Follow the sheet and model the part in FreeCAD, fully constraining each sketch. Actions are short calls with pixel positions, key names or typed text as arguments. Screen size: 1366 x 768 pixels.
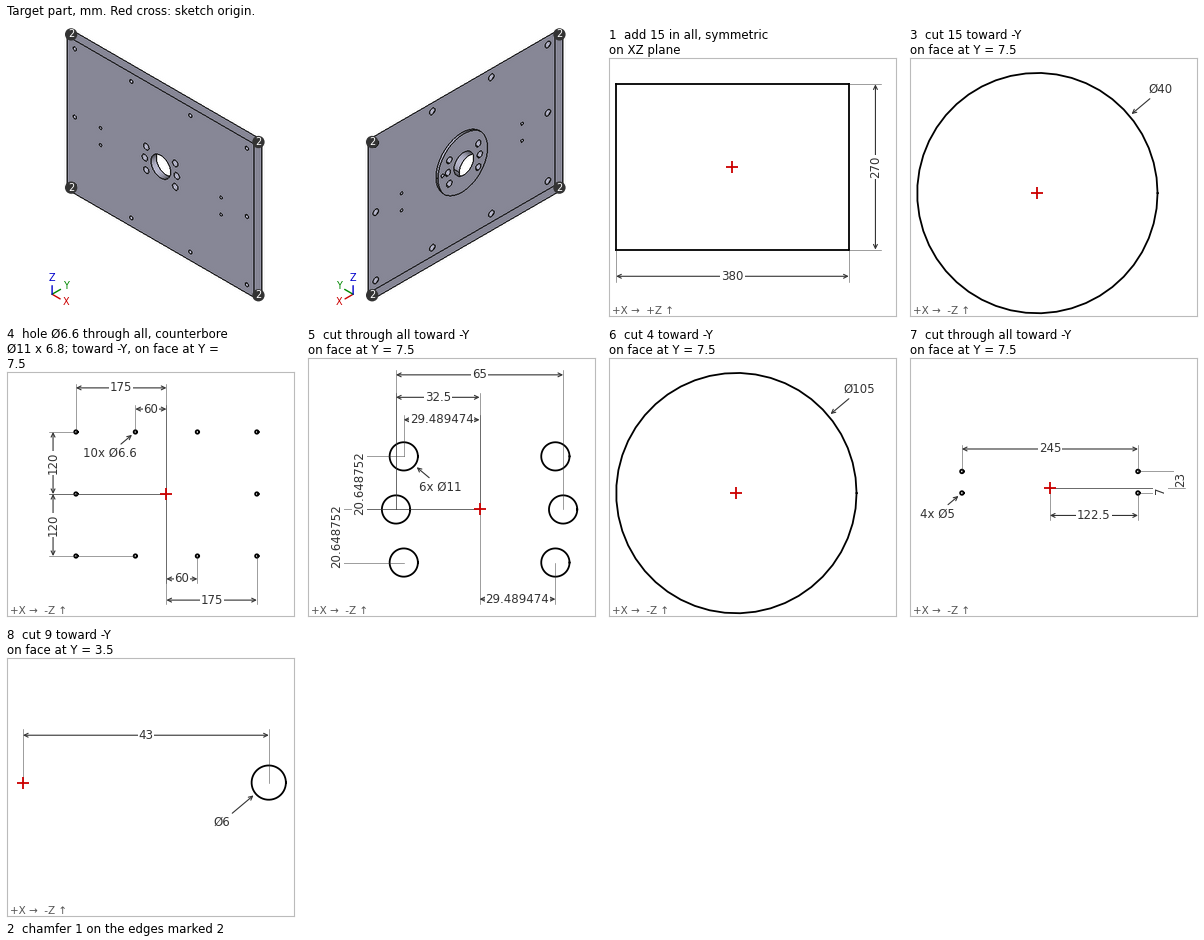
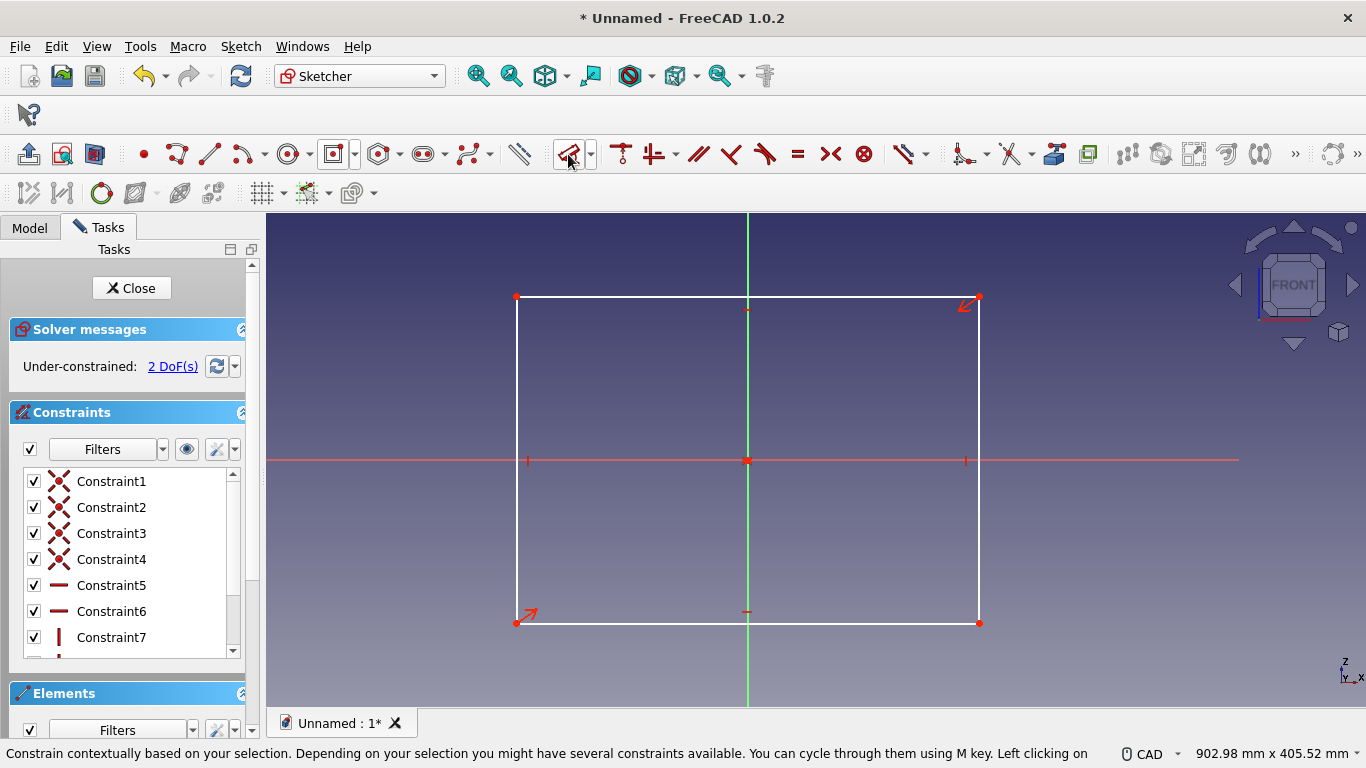
click(655, 624)
click(641, 658)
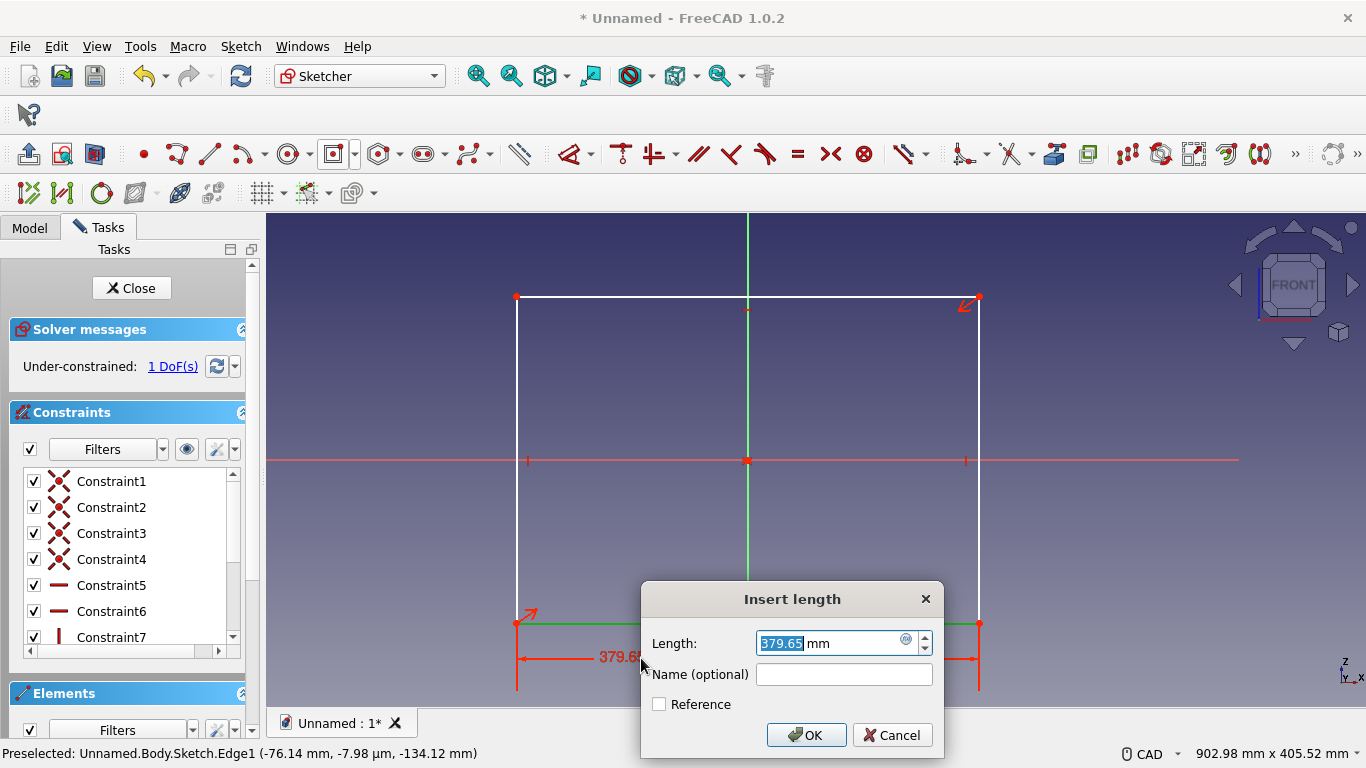
text(380)
key(Return)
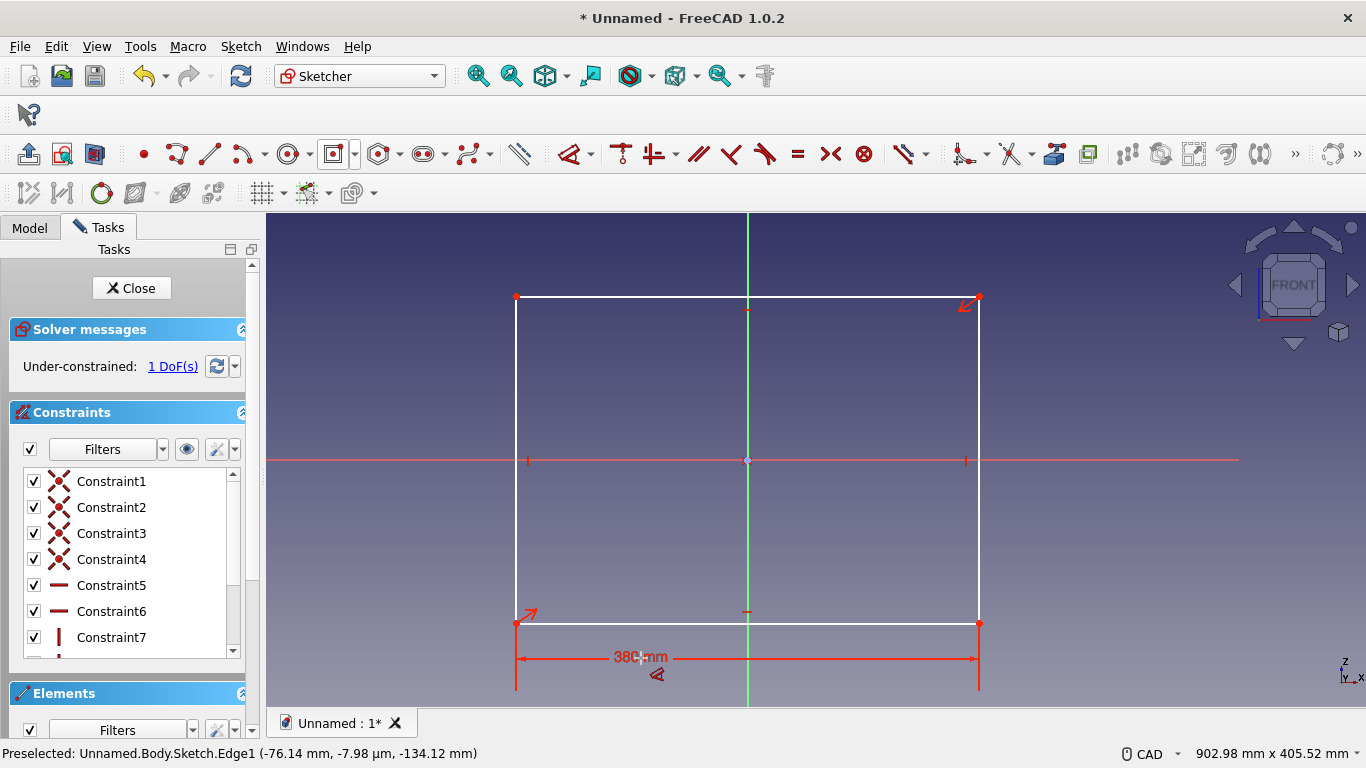
click(979, 526)
click(1013, 385)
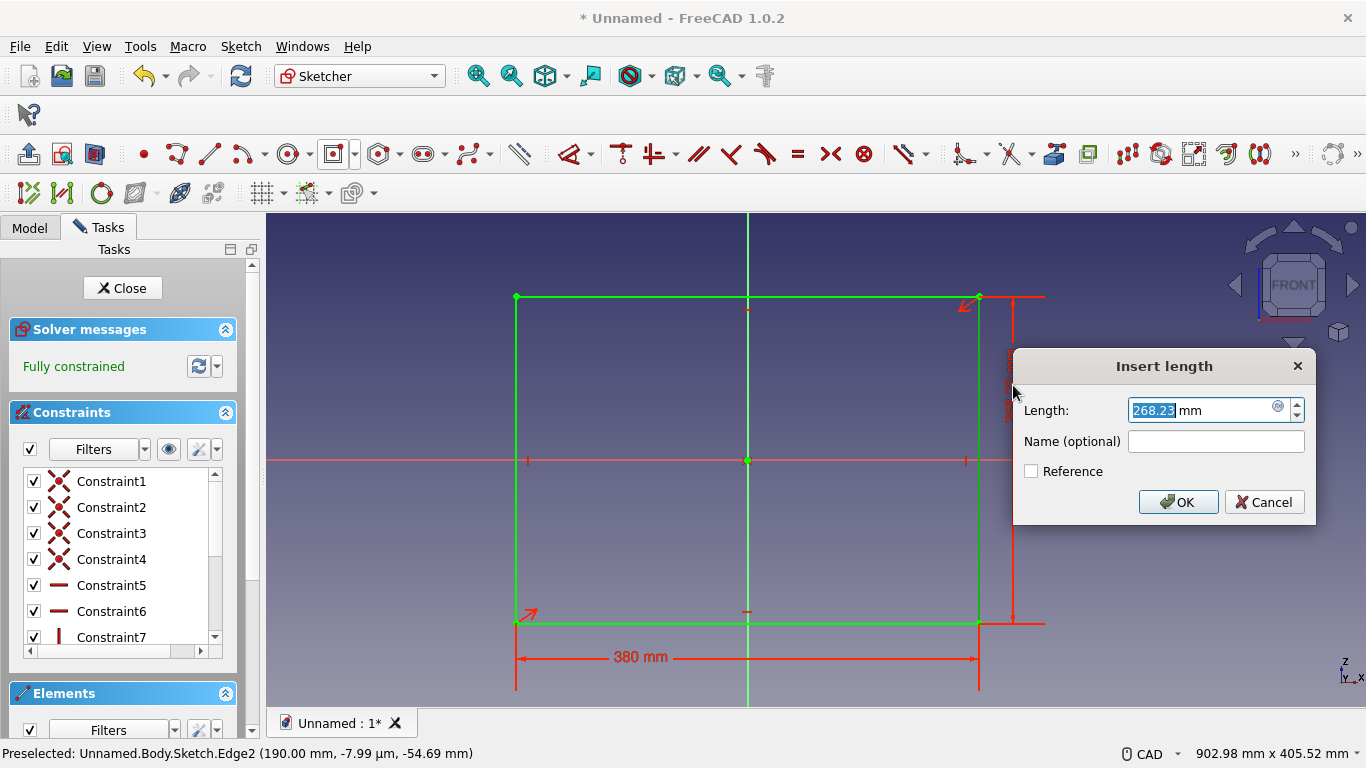
text(270)
key(Return)
key(Escape)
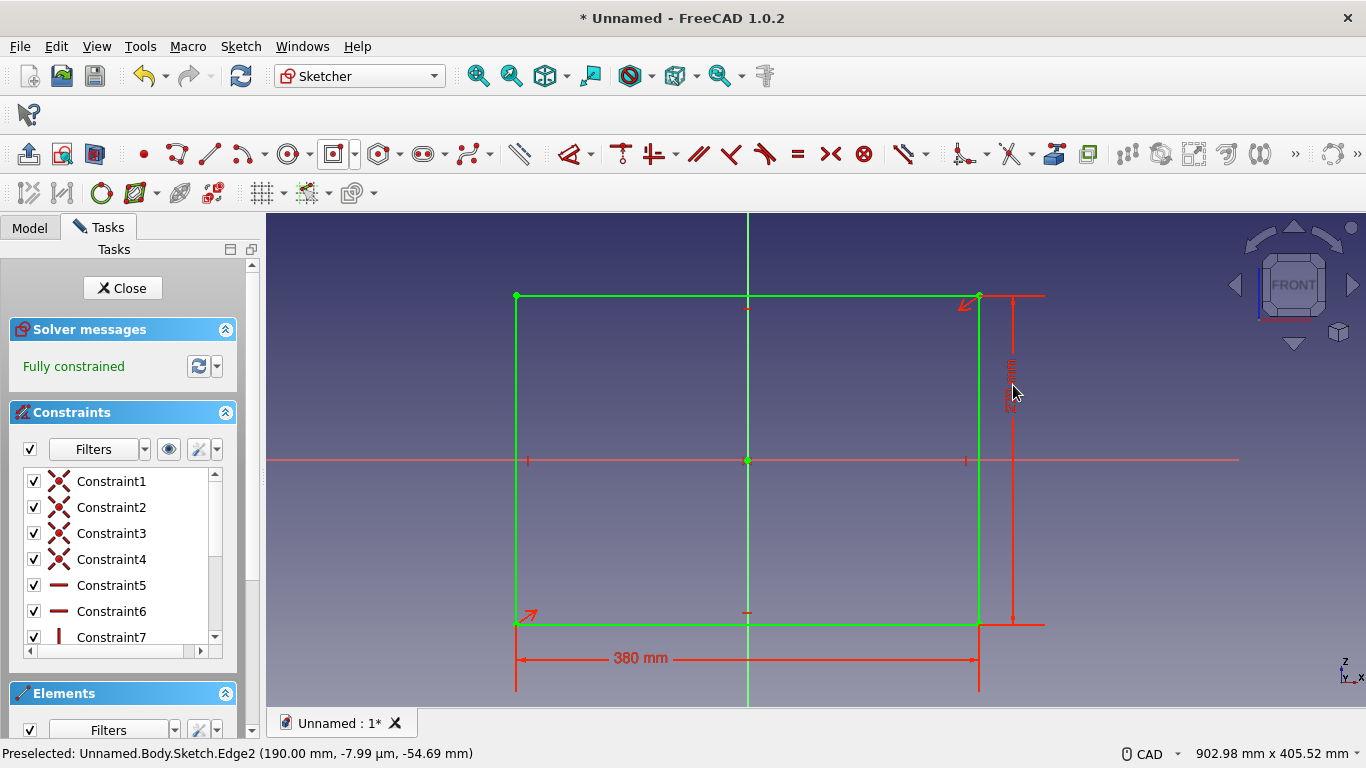
click(123, 288)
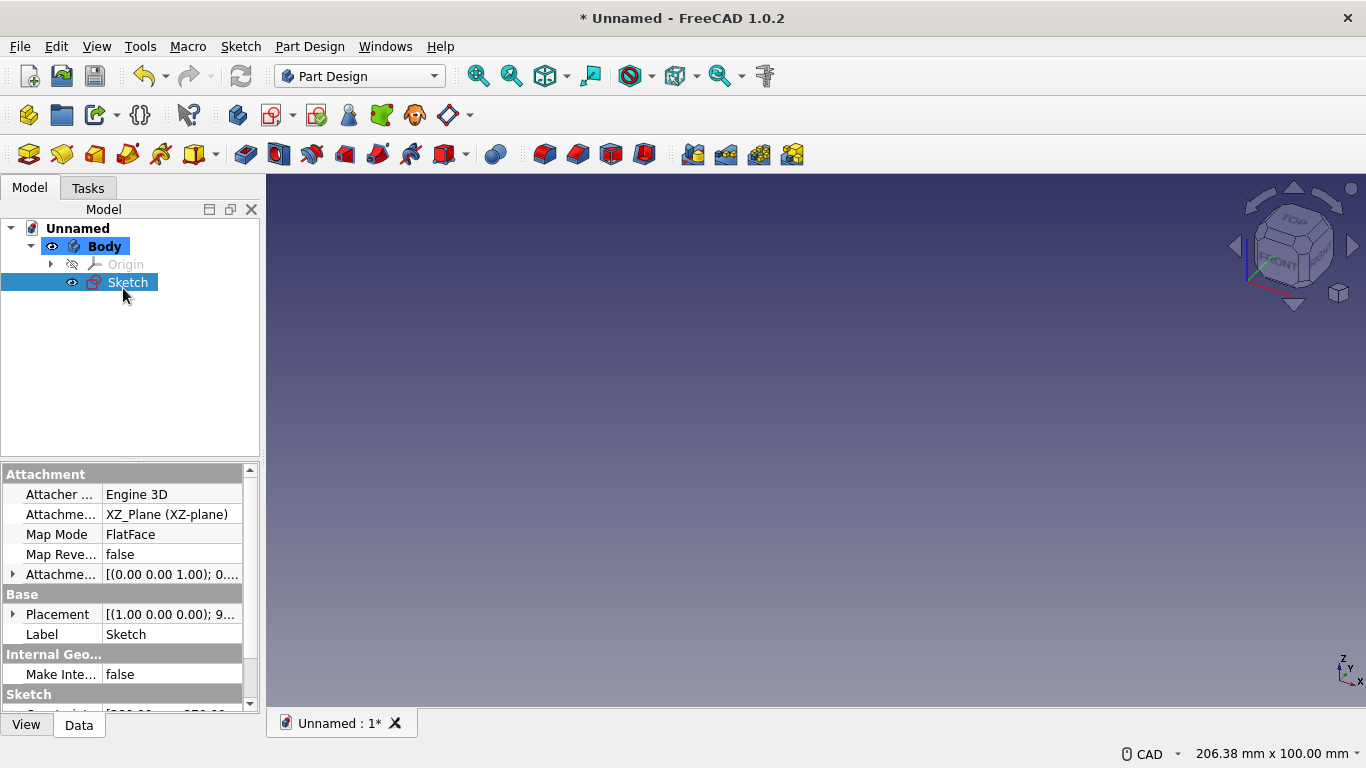
click(29, 154)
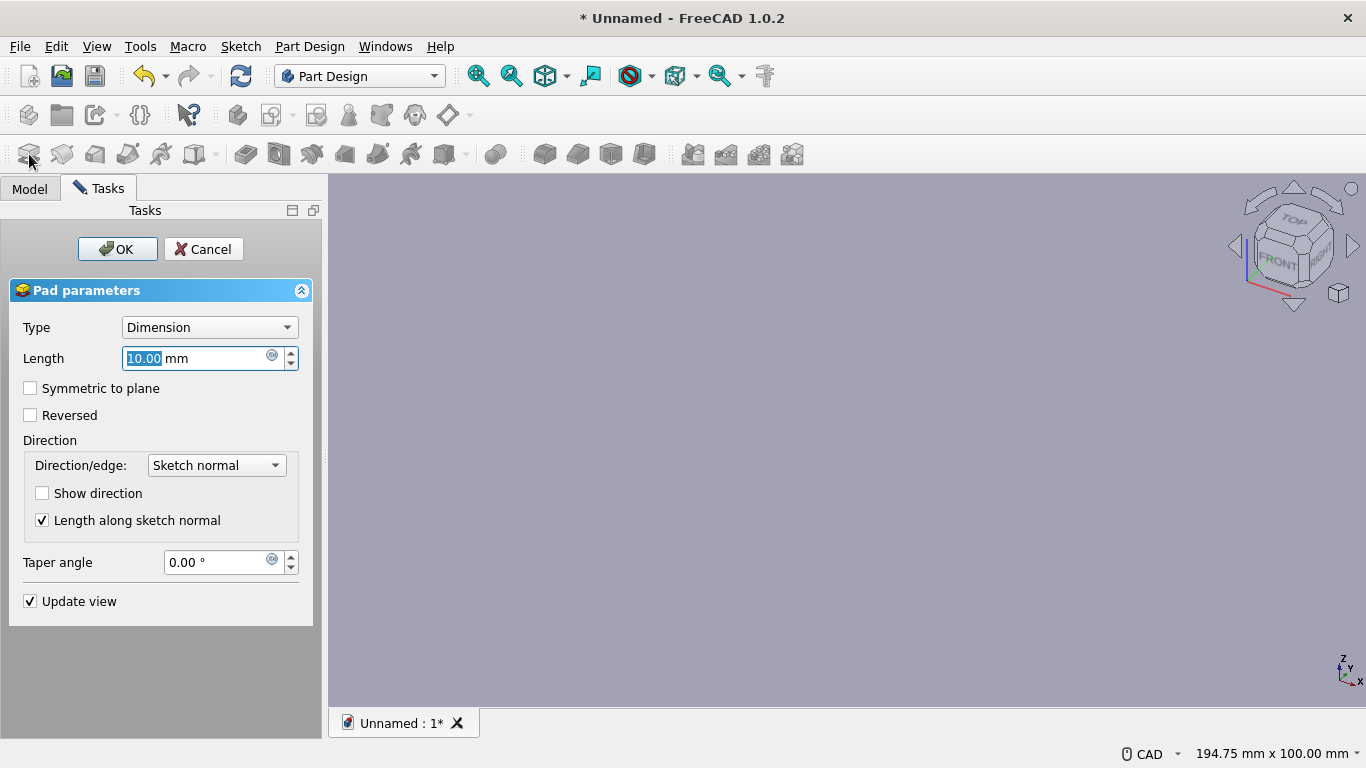
text(15)
key(Tab)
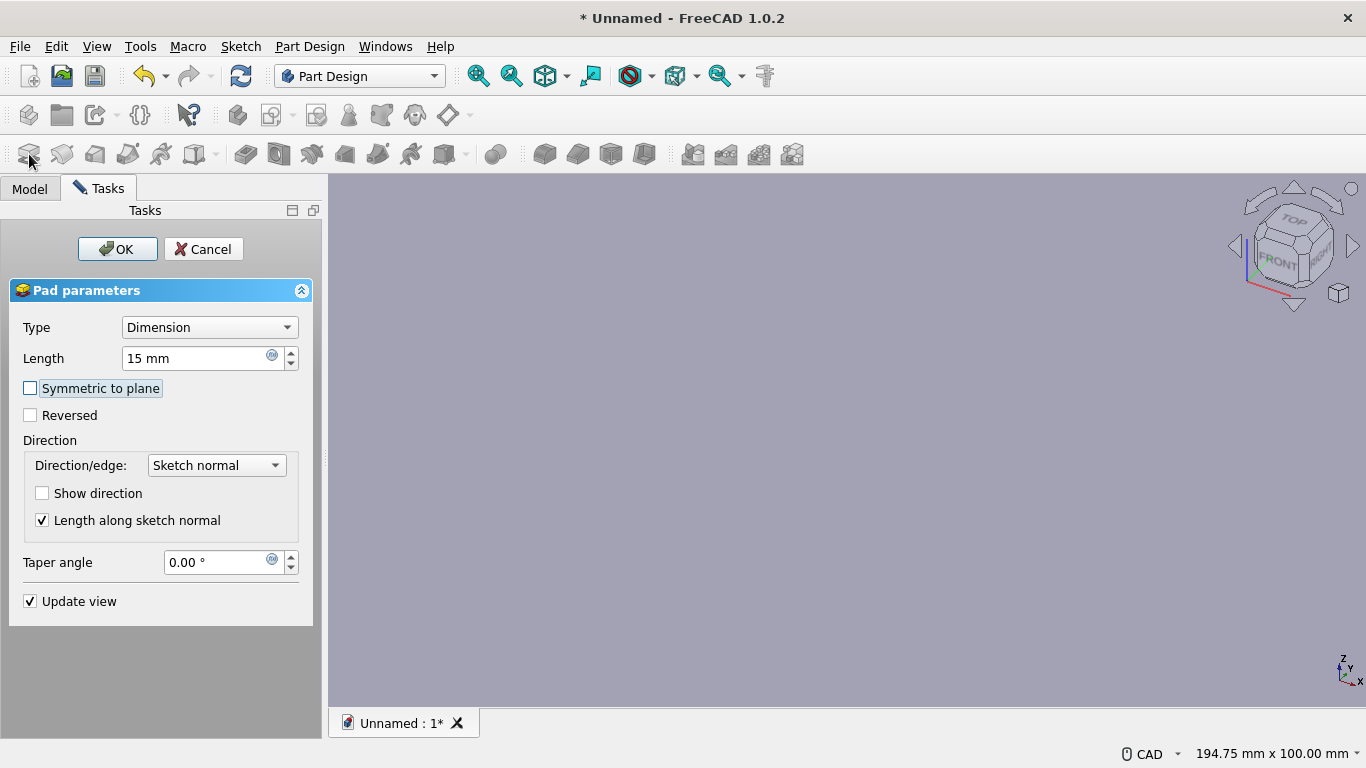
click(31, 388)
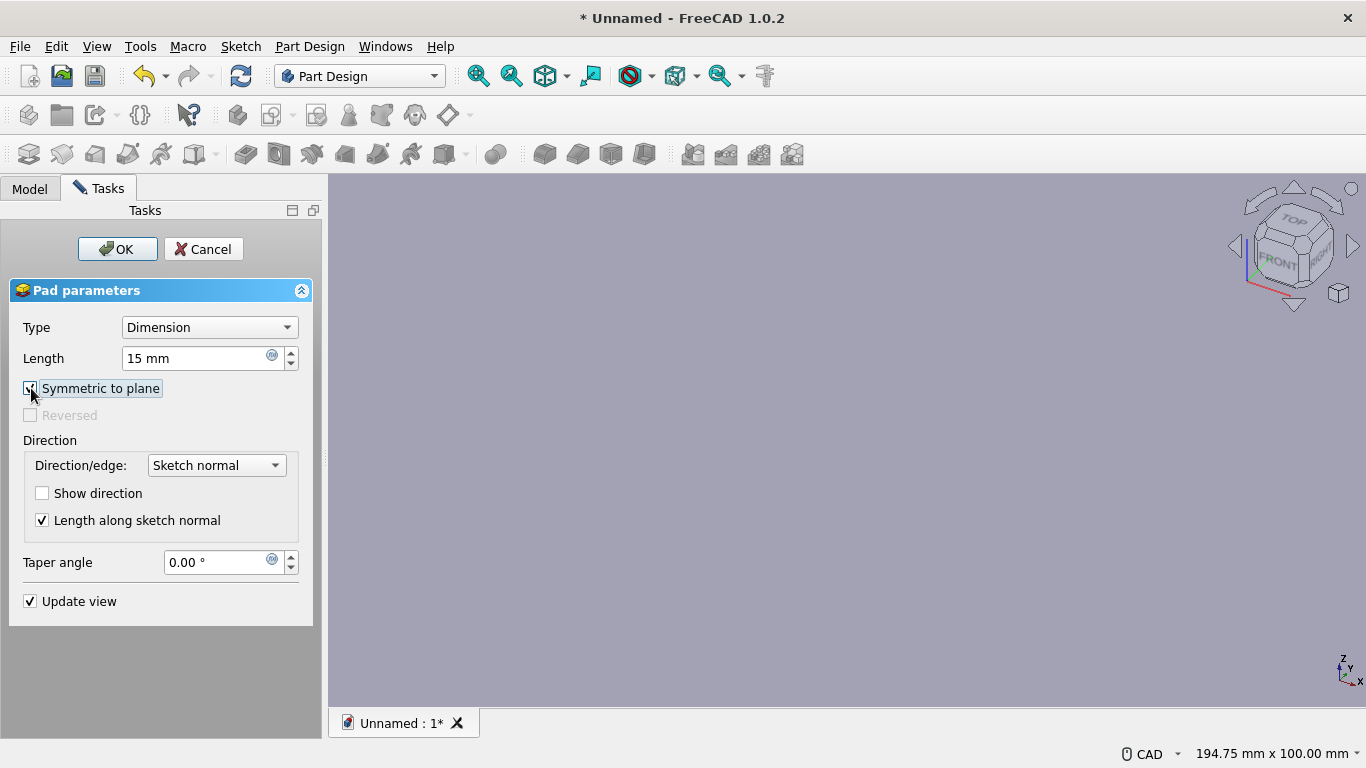
click(118, 249)